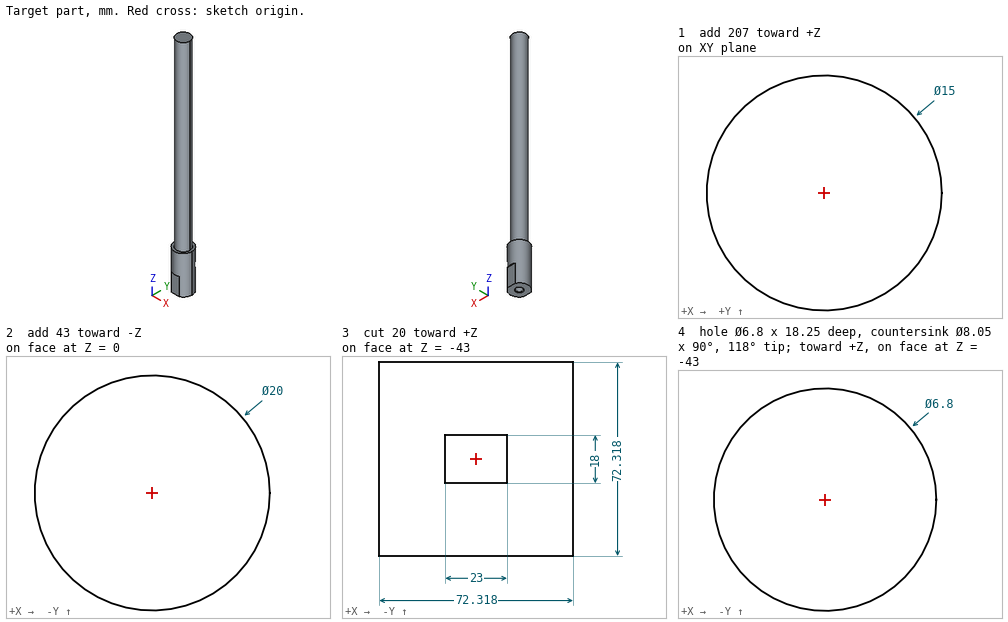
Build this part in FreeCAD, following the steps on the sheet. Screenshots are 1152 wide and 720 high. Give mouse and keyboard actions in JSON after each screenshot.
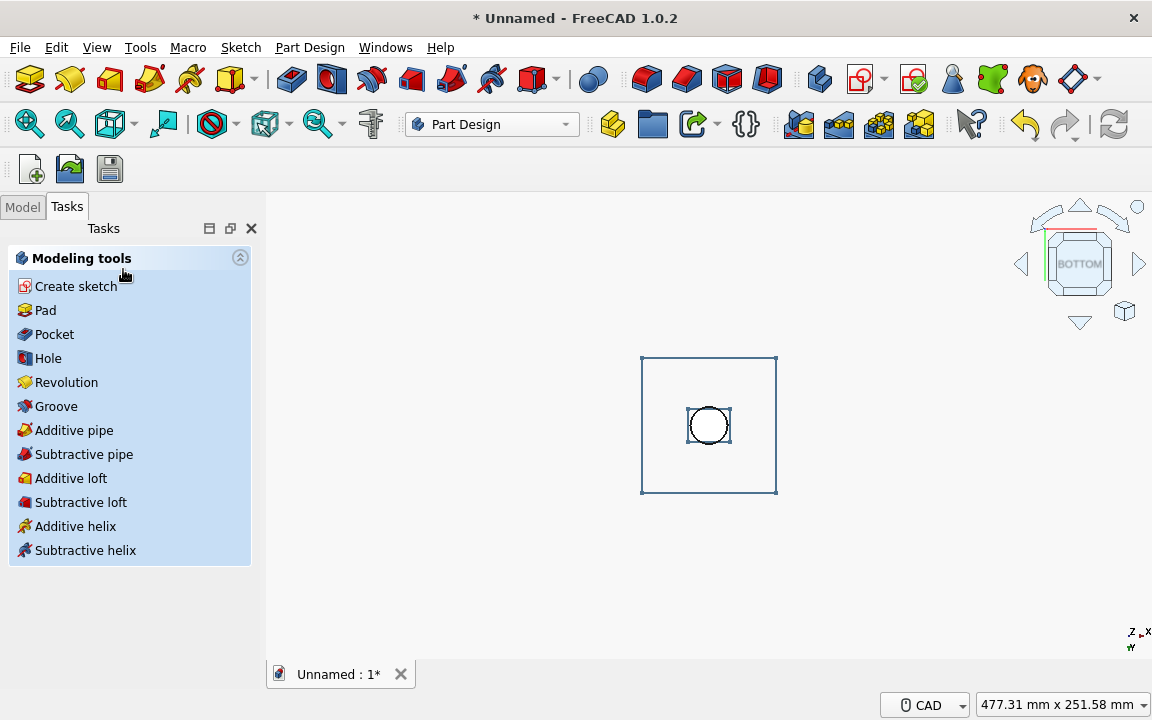
{"action": "left_click", "coordinate": [292, 80]}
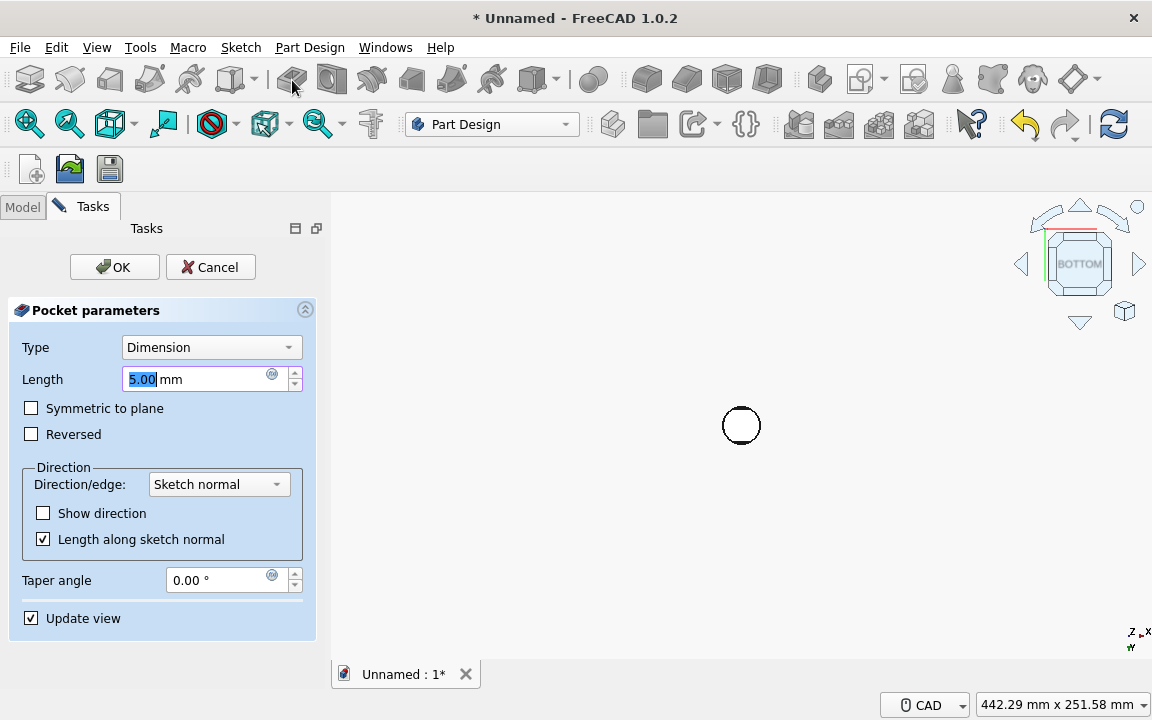
{"action": "type", "text": "20"}
{"action": "key", "text": "Tab"}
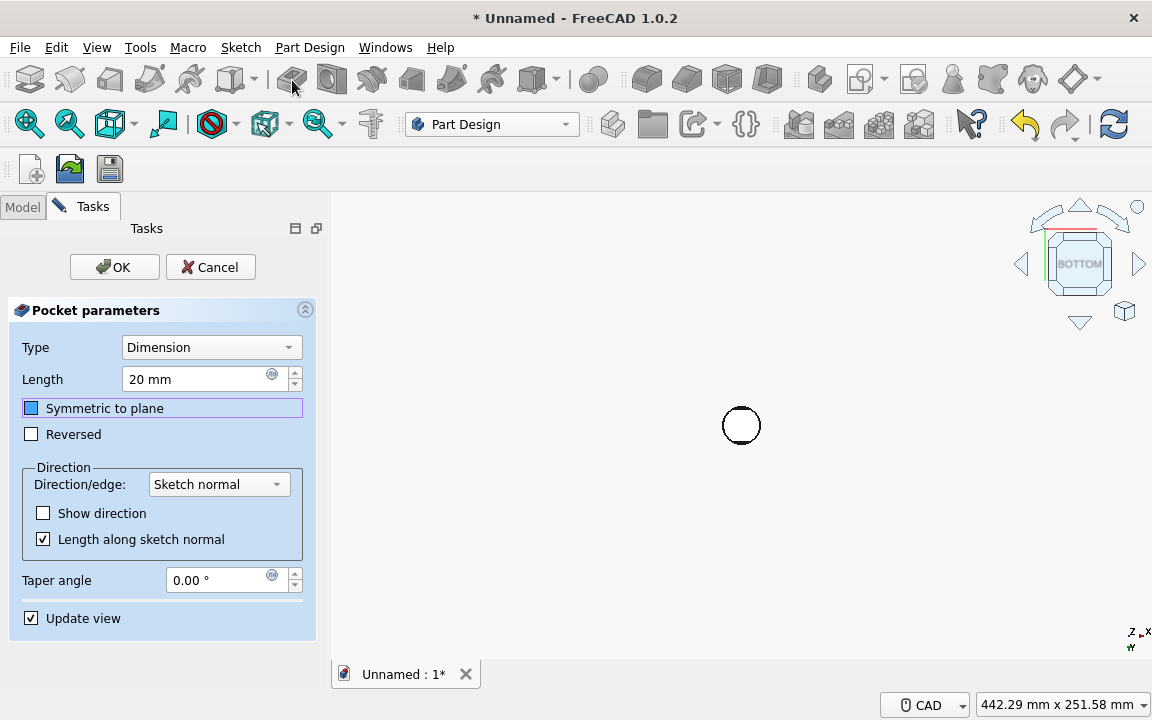
{"action": "left_click", "coordinate": [115, 267]}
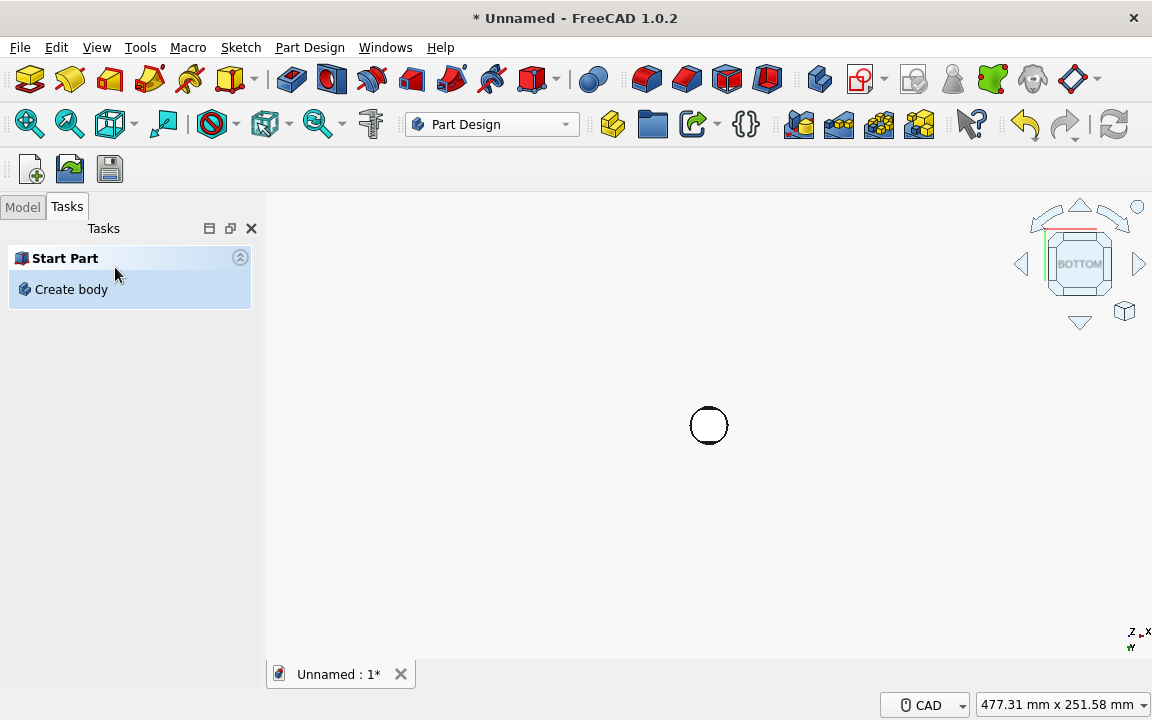
{"action": "left_click", "coordinate": [30, 124]}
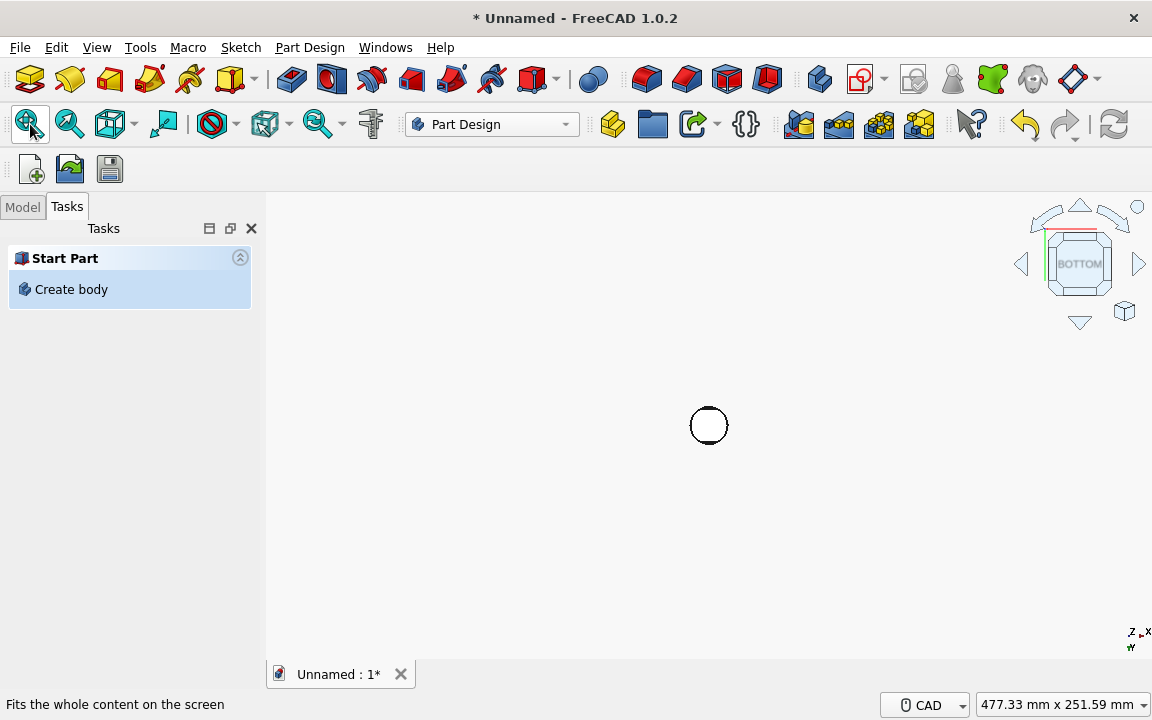
{"action": "left_click", "coordinate": [709, 424]}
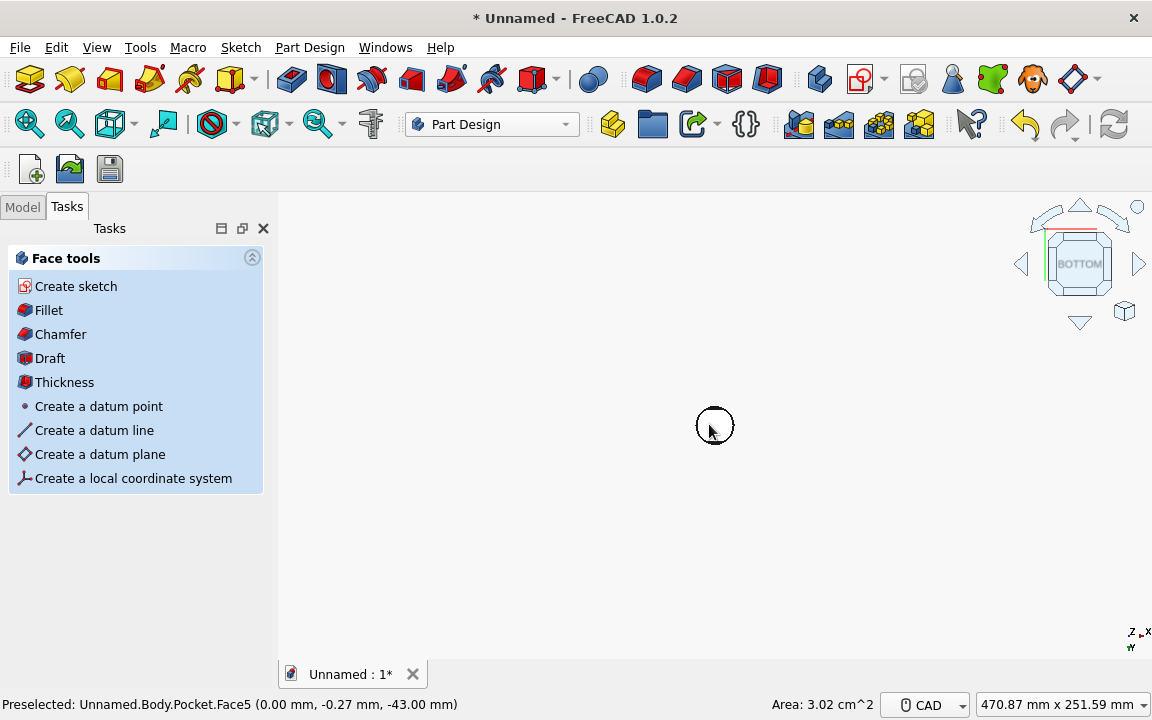
{"action": "left_click", "coordinate": [860, 80]}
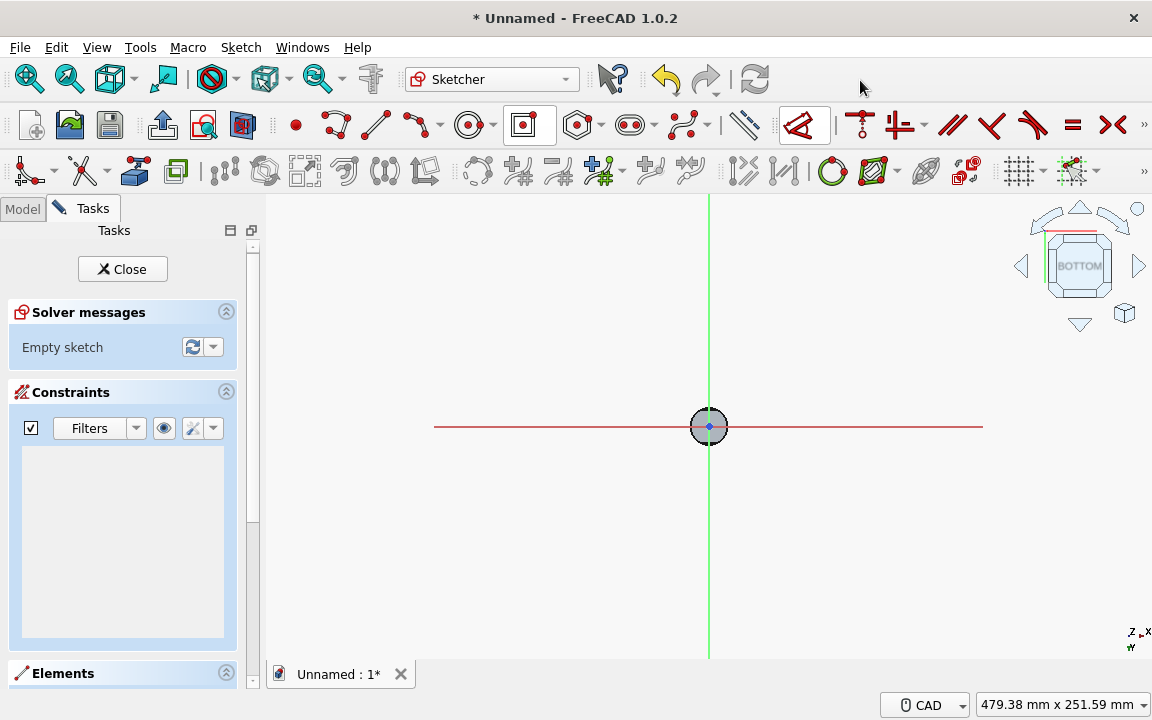
{"action": "scroll", "coordinate": [713, 426], "scroll_direction": "up", "scroll_amount": 15}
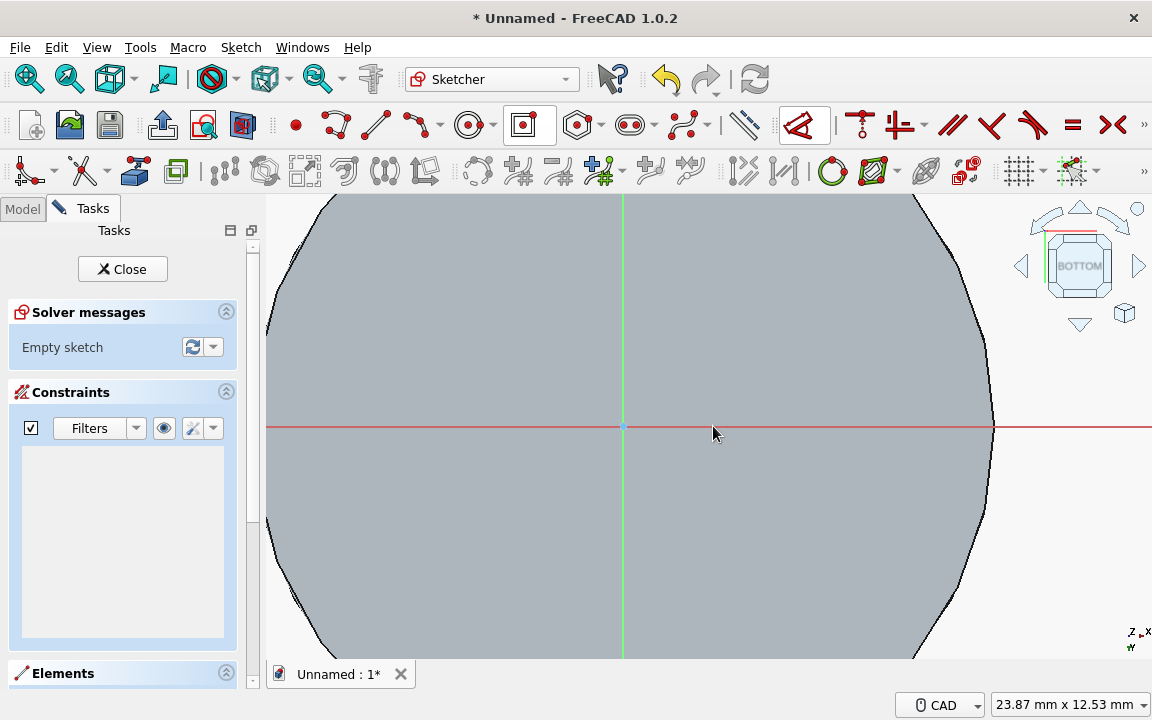
{"action": "key", "text": "g c"}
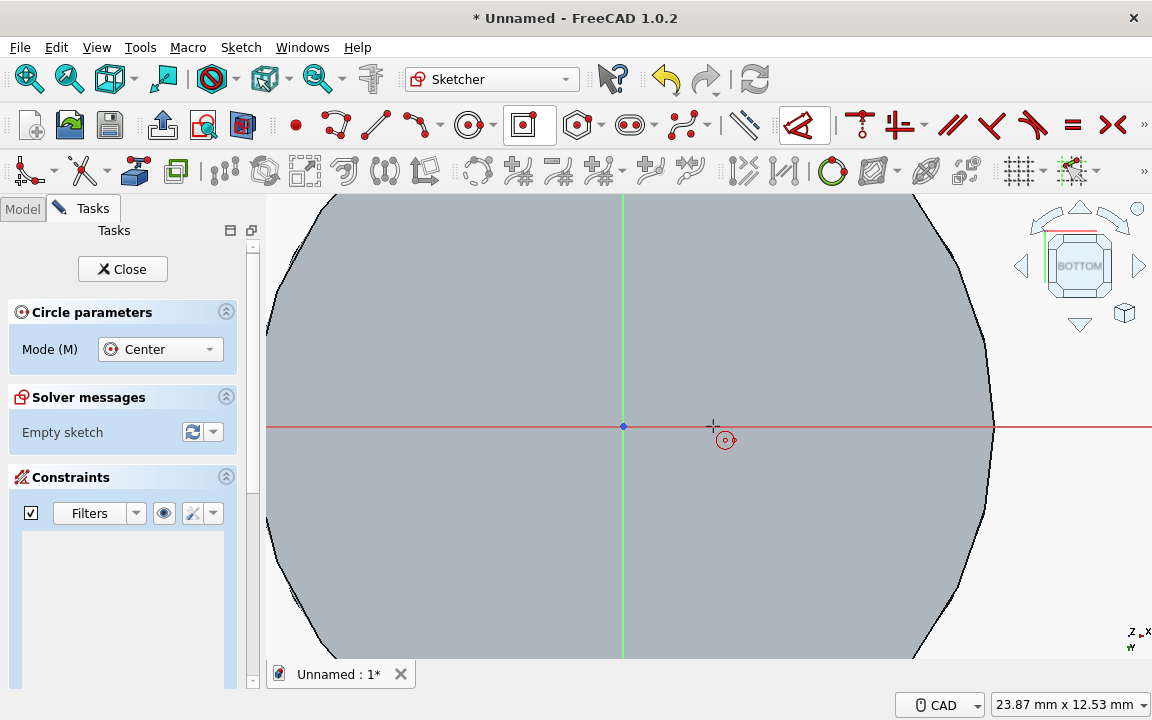
{"action": "left_click", "coordinate": [623, 426]}
{"action": "mouse_move", "coordinate": [712, 337]}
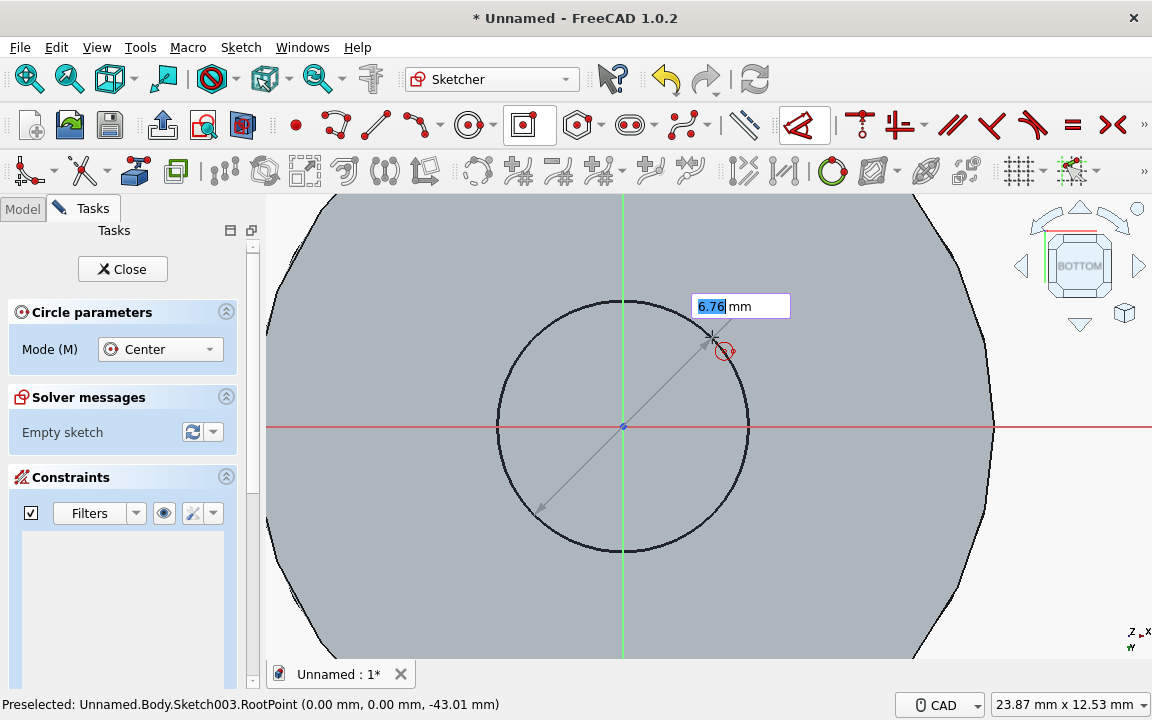
{"action": "type", "text": "6.8"}
{"action": "key", "text": "Return"}
{"action": "key", "text": "Escape"}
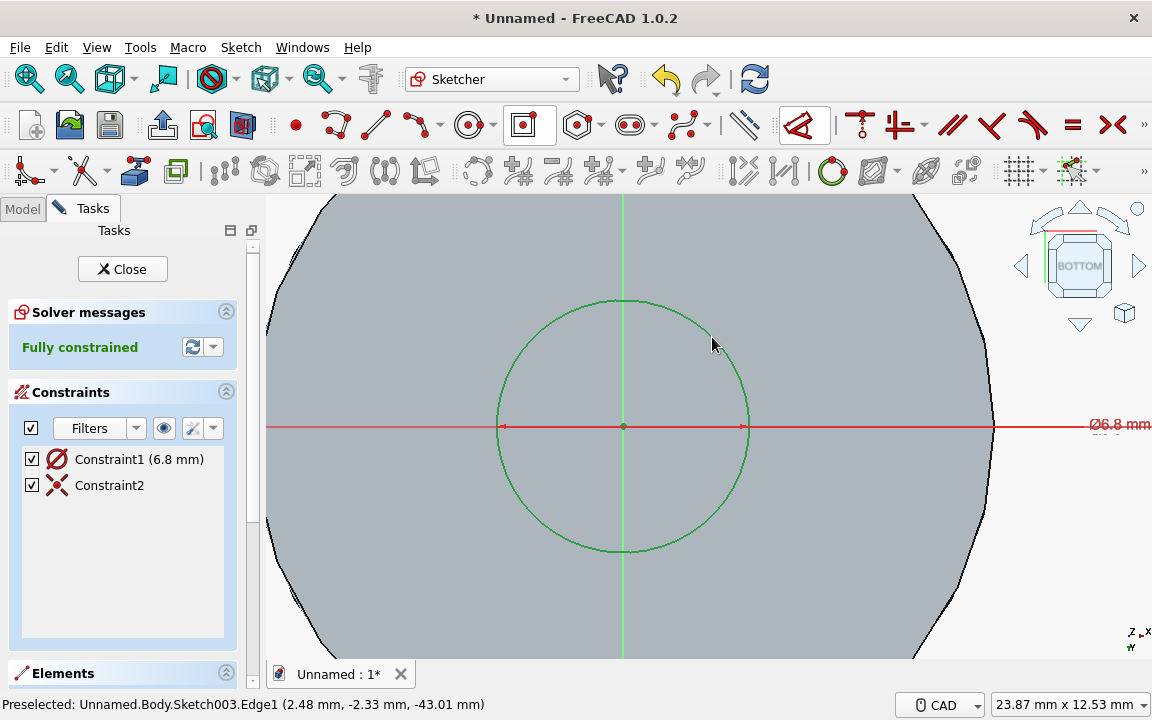
{"action": "left_click", "coordinate": [123, 269]}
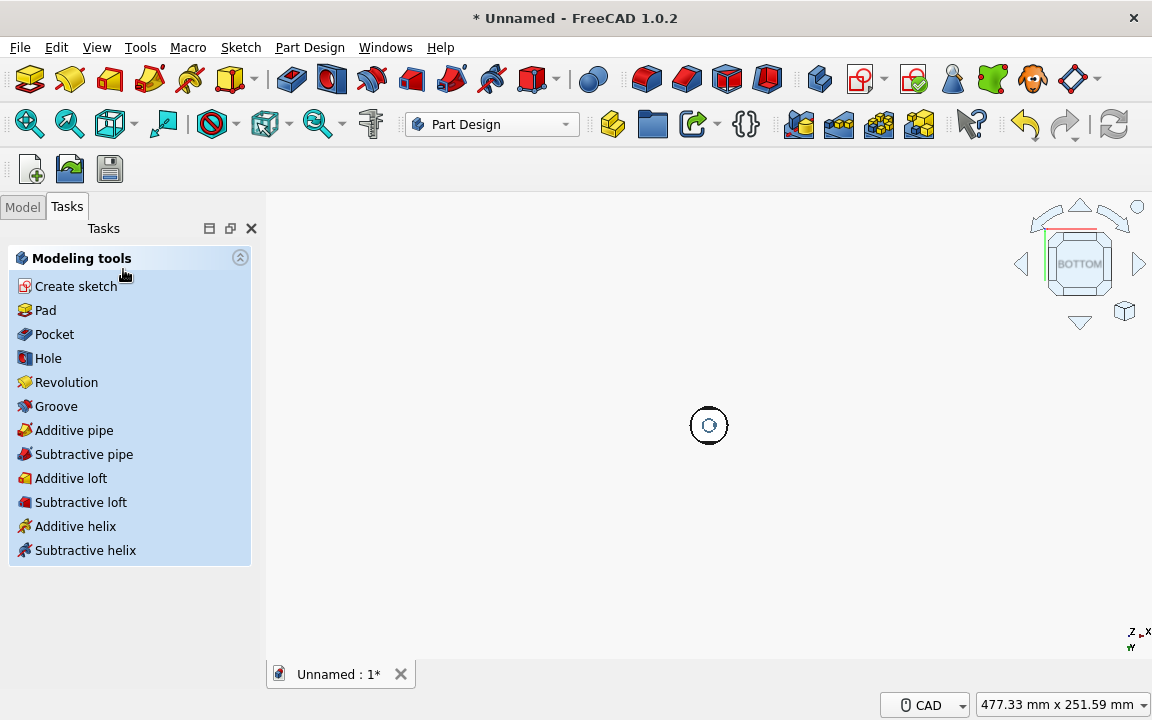
{"action": "left_click", "coordinate": [332, 80]}